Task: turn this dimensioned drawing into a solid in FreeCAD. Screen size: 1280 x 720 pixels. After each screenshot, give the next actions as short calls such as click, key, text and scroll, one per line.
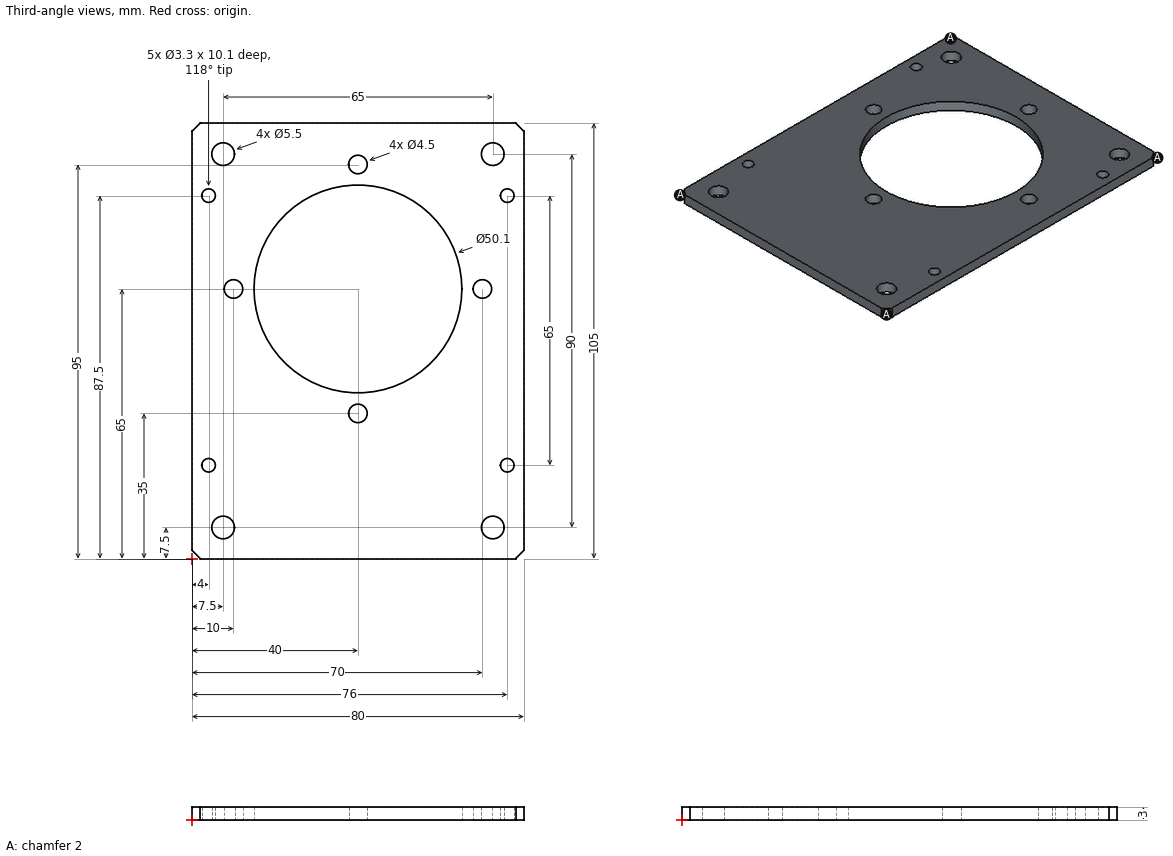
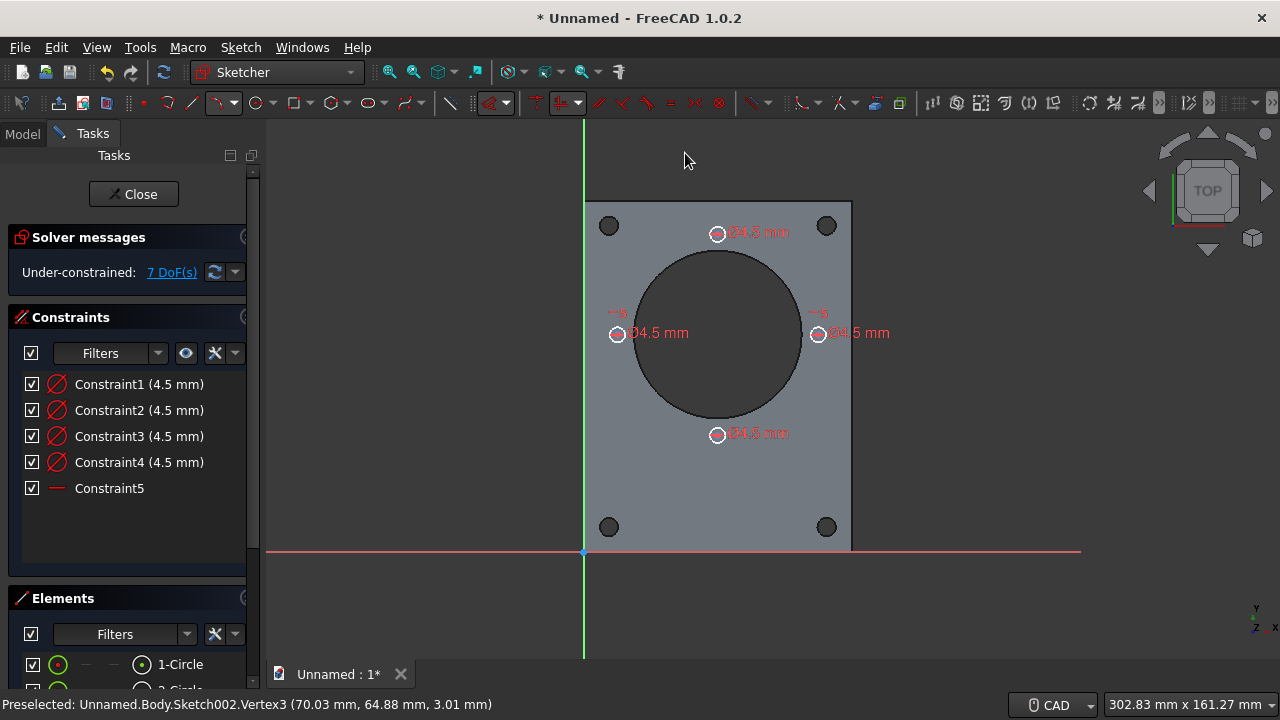
click(718, 234)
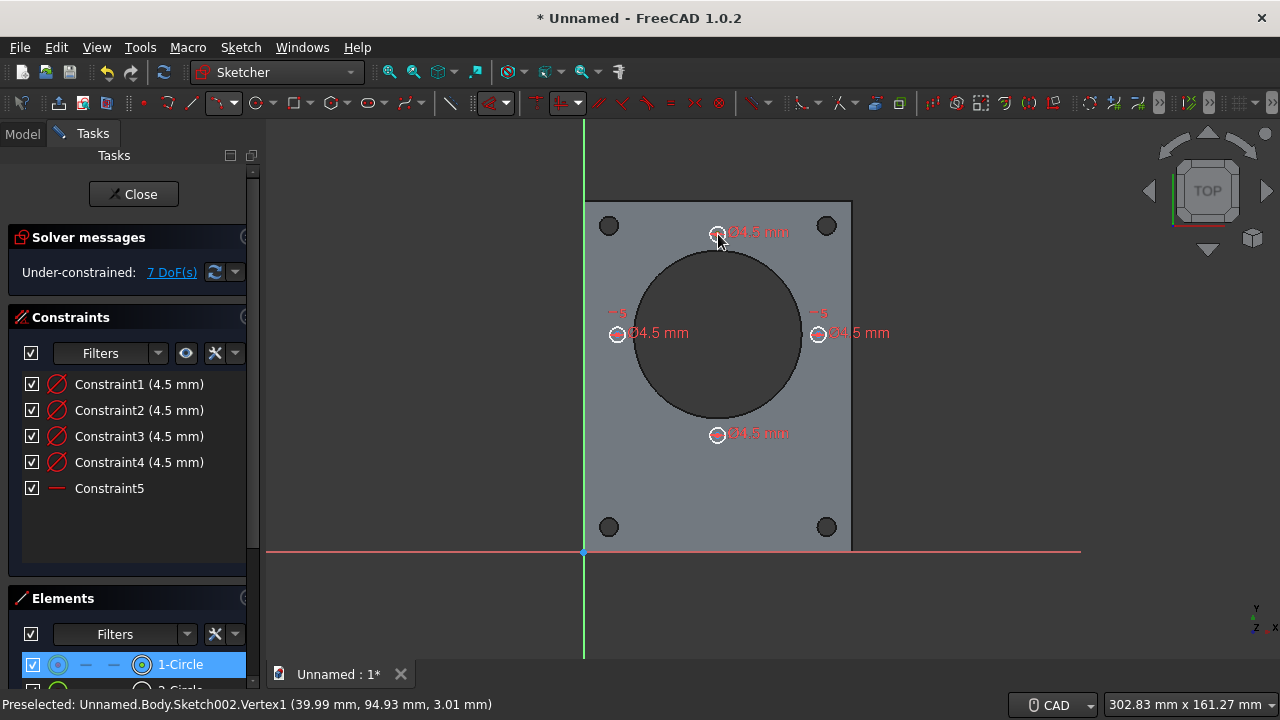
click(718, 435)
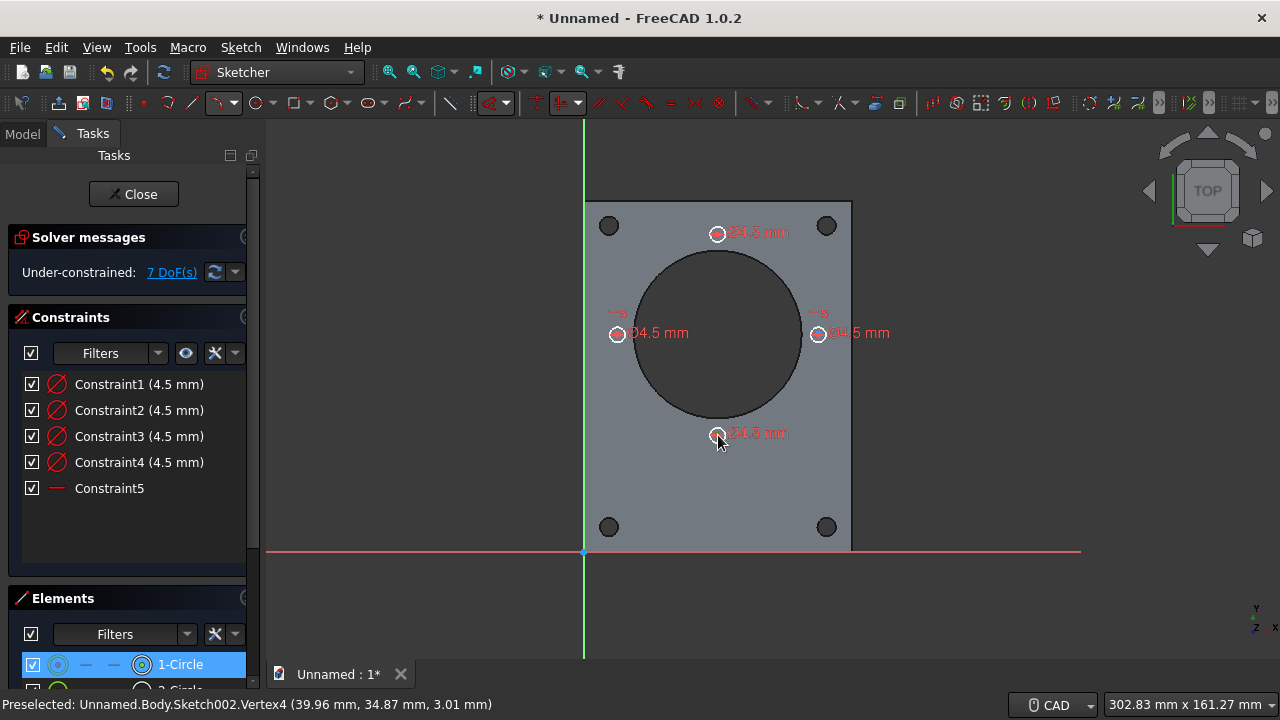
click(580, 104)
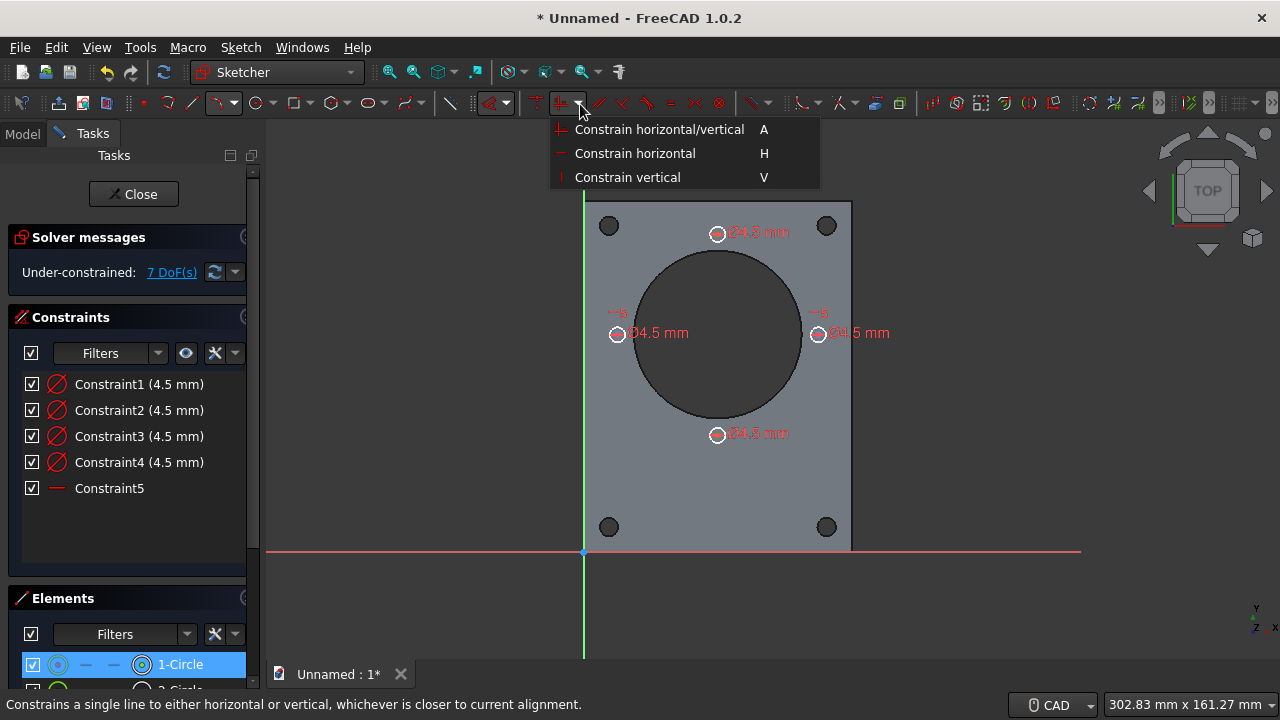
click(685, 177)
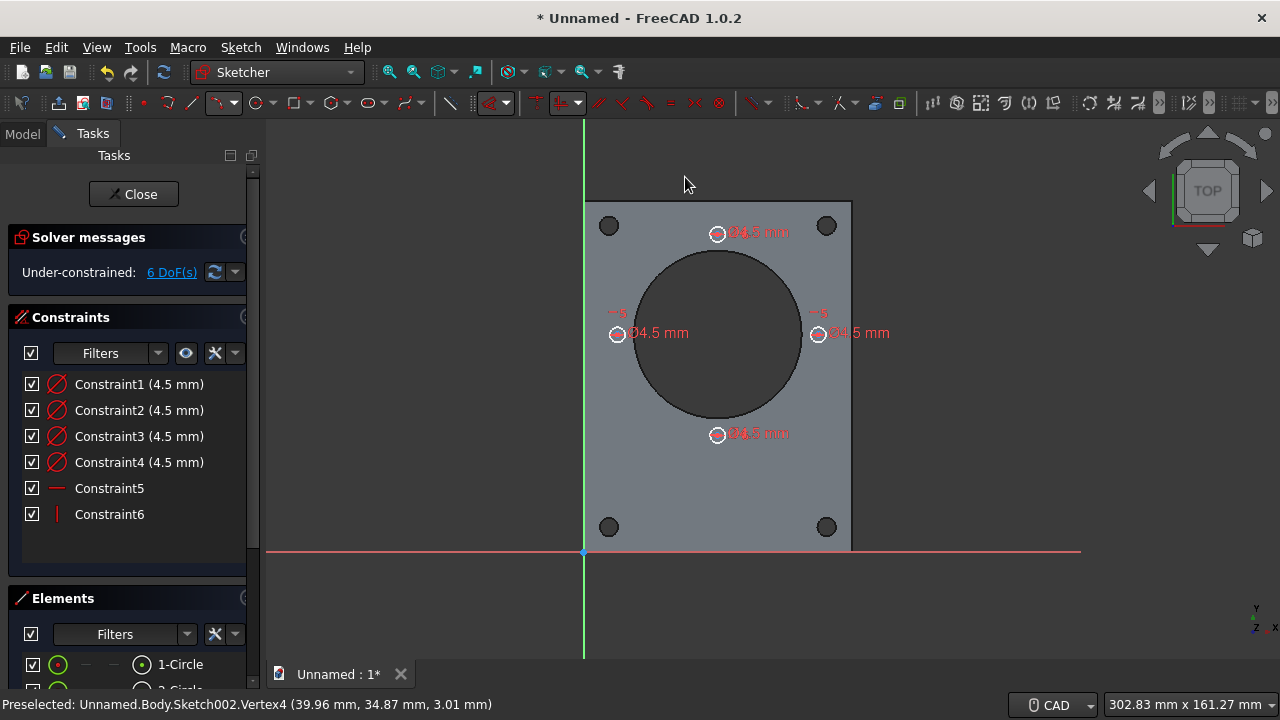
click(718, 234)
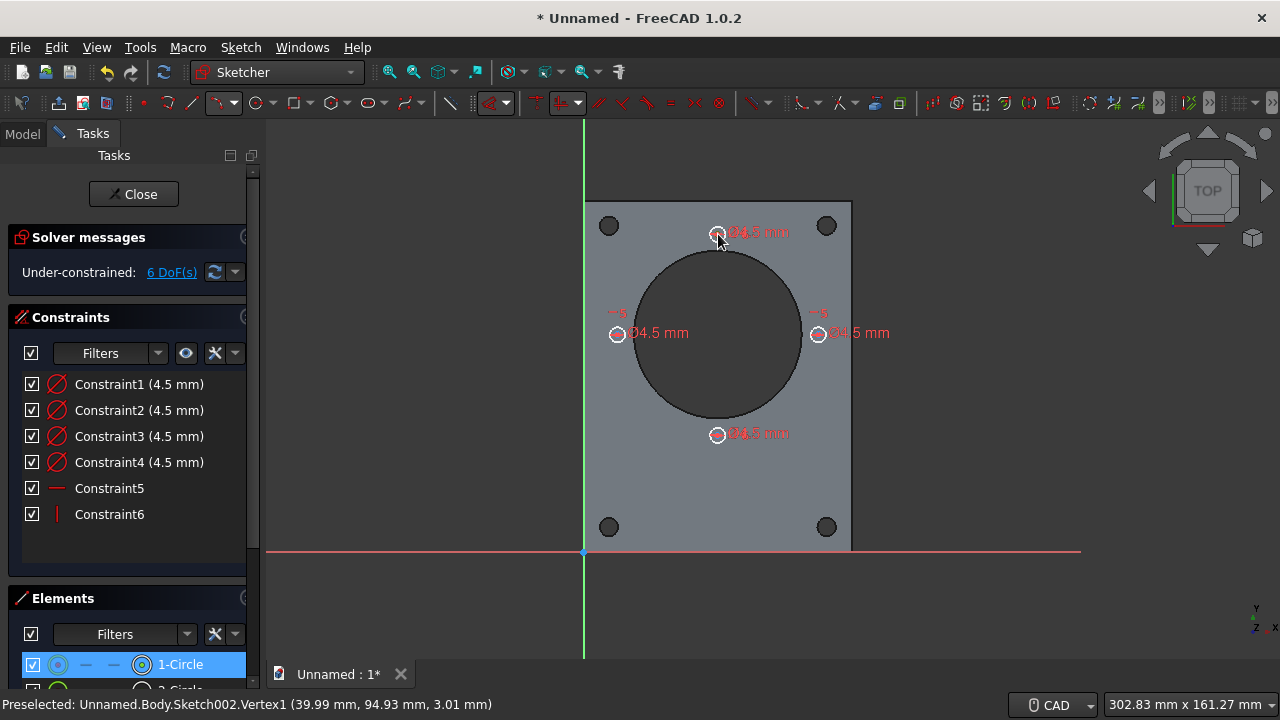
key(l)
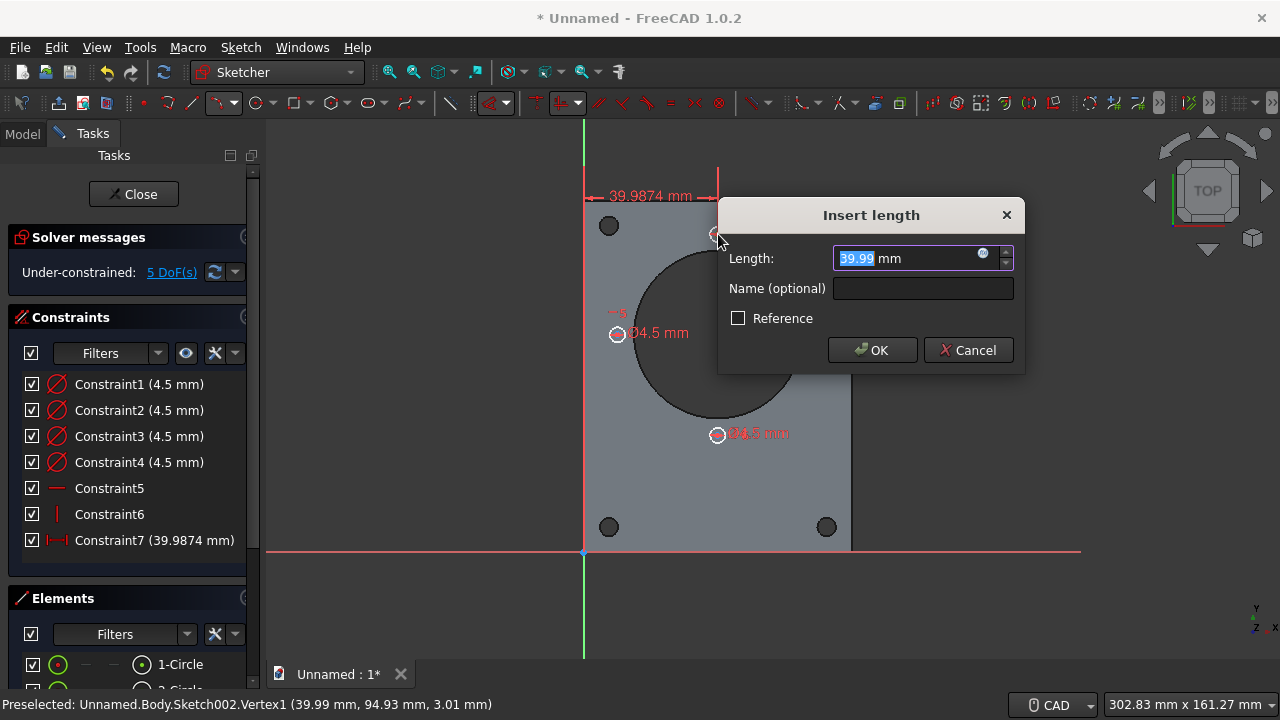
text(40)
key(Return)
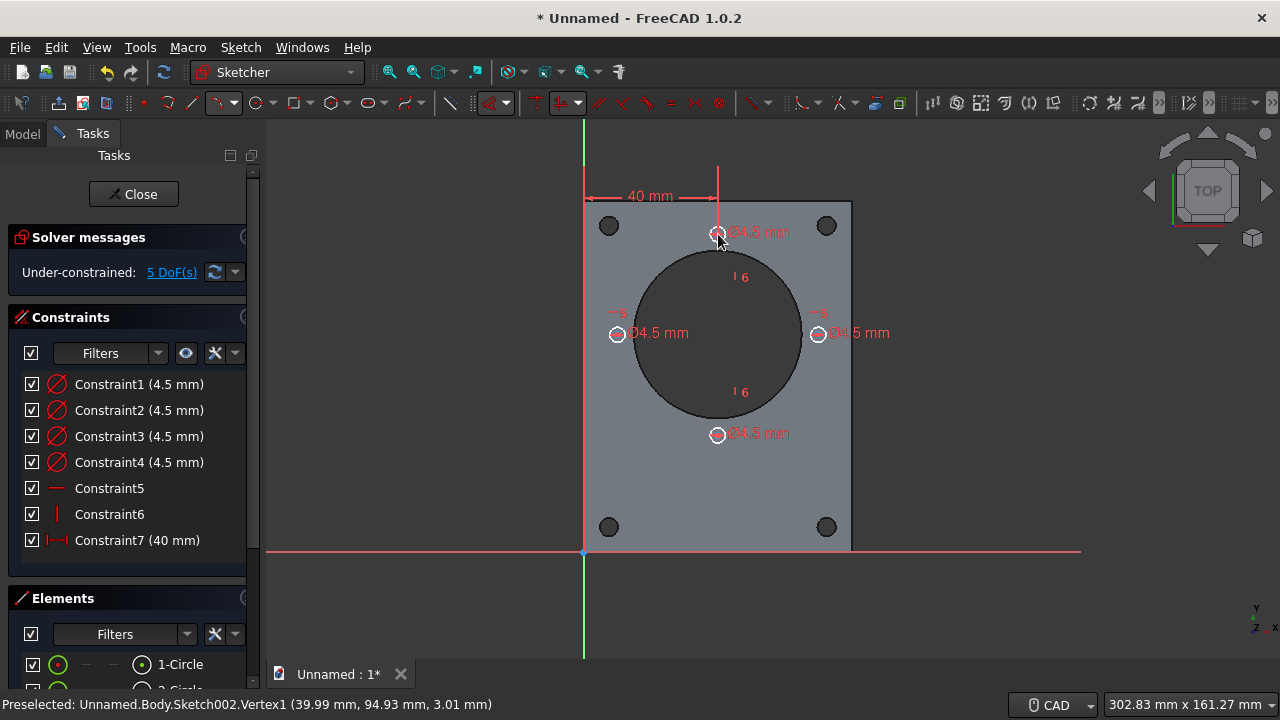
click(718, 234)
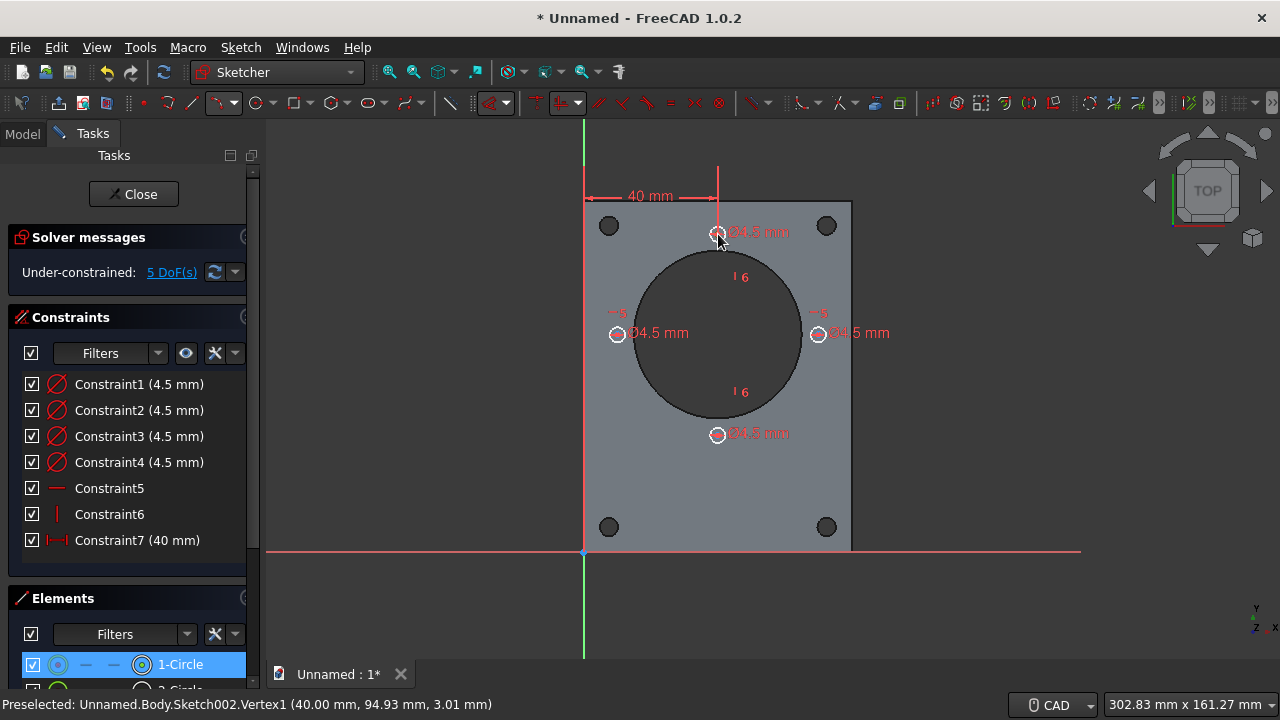
key(i)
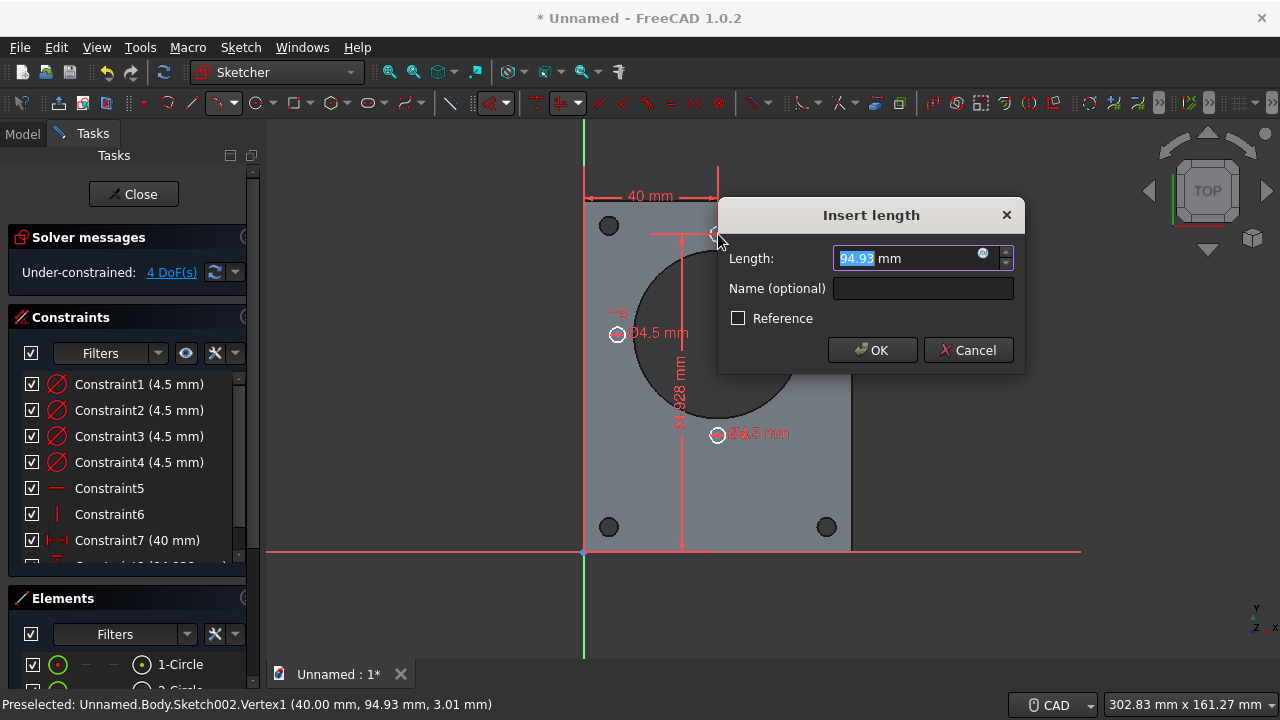
text(95)
key(Return)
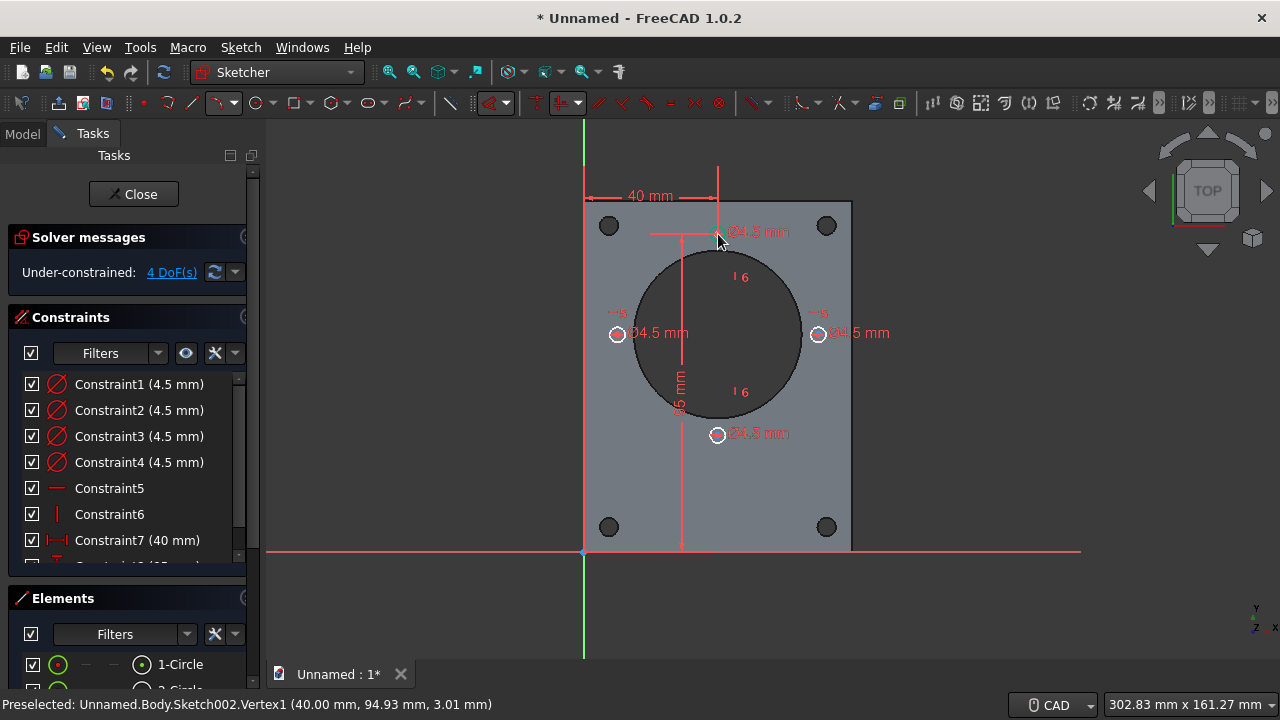
click(617, 335)